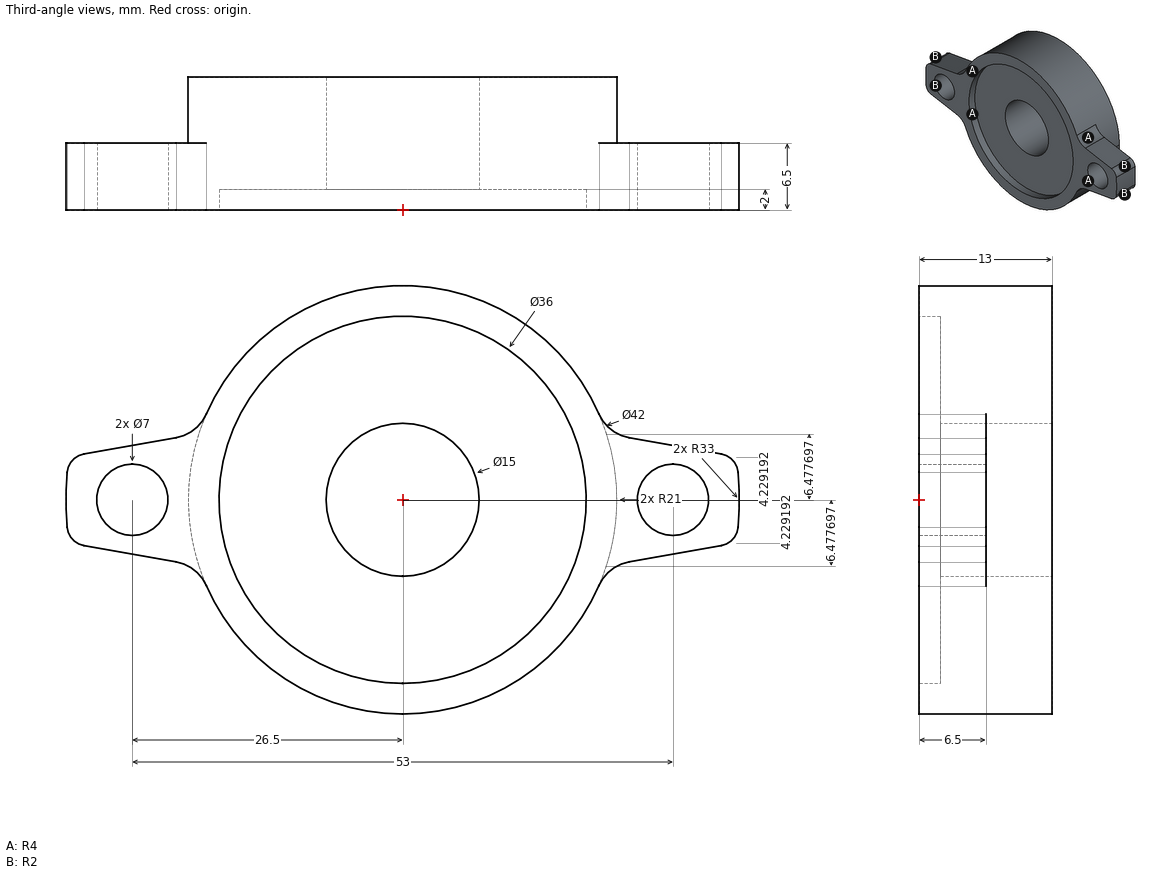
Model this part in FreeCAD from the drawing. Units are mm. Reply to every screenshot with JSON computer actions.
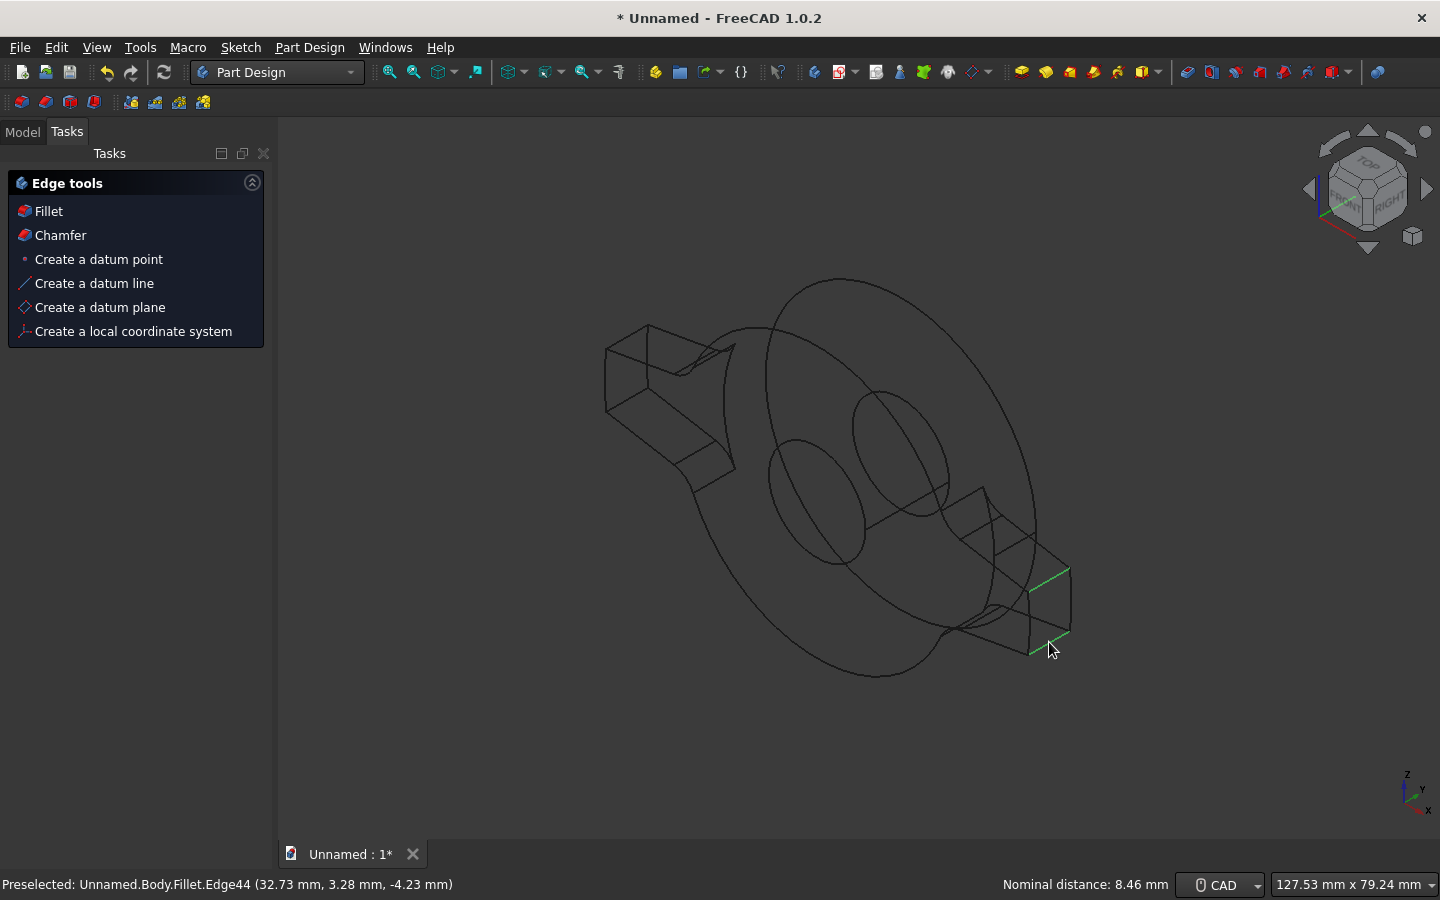
{"action": "left_click", "coordinate": [627, 399], "text": "ctrl"}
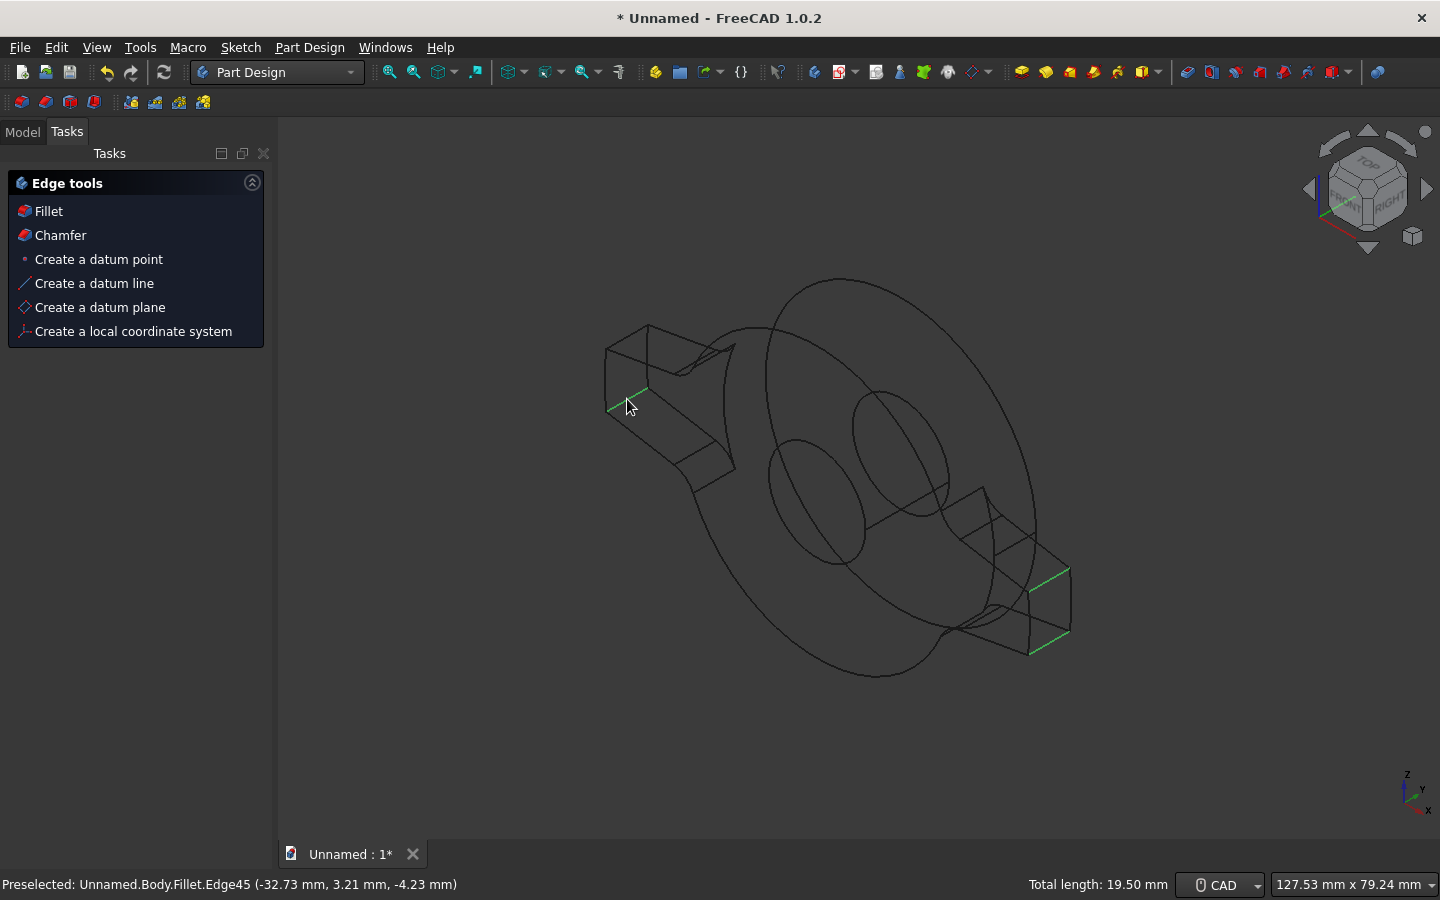
{"action": "left_click", "coordinate": [627, 336], "text": "ctrl"}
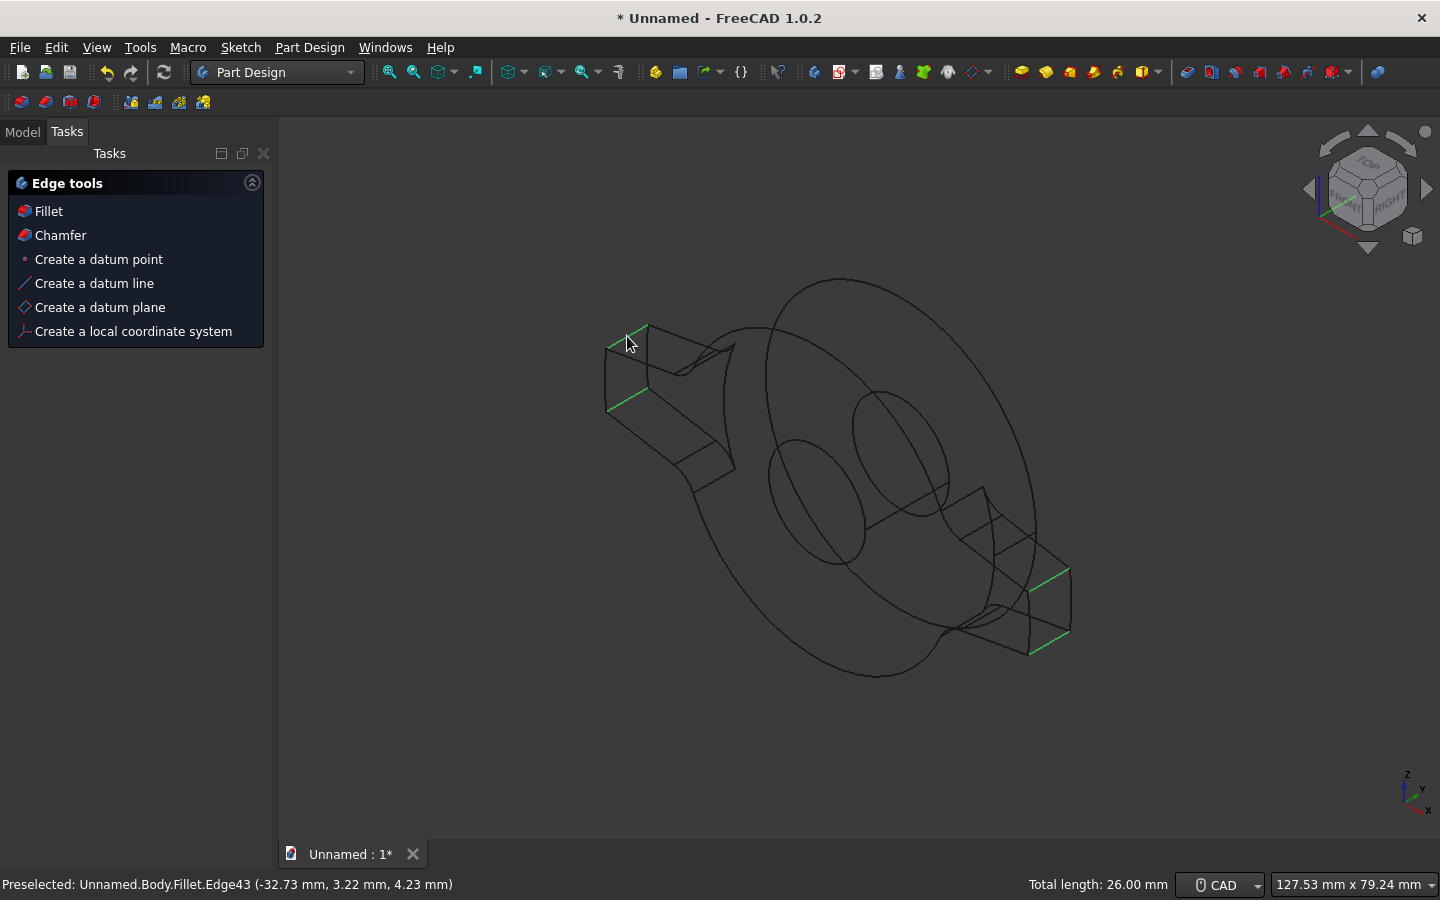
{"action": "key", "text": "v 1"}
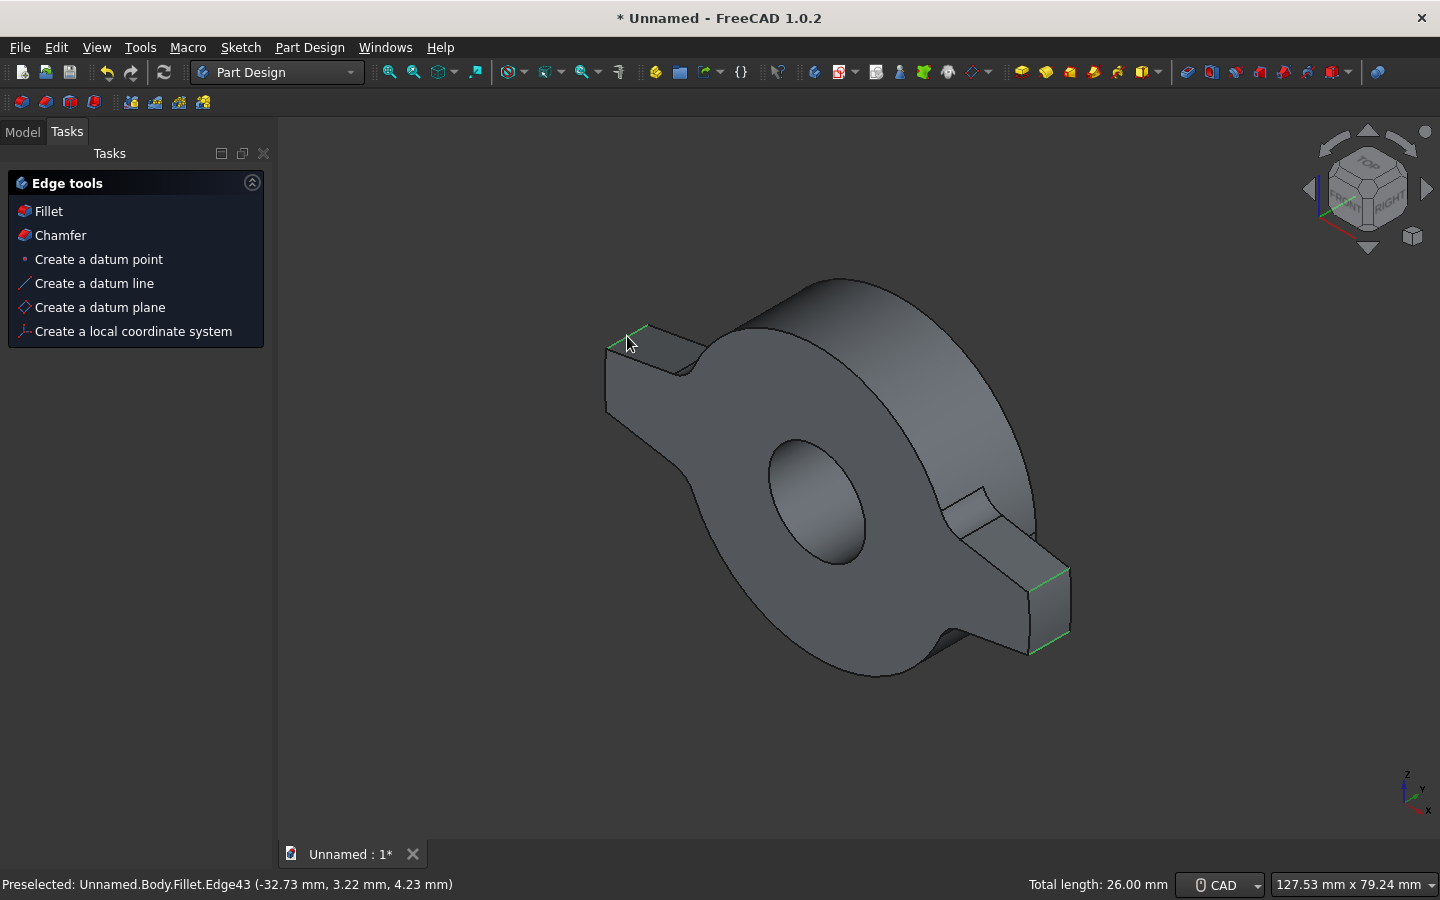
{"action": "left_click", "coordinate": [22, 102]}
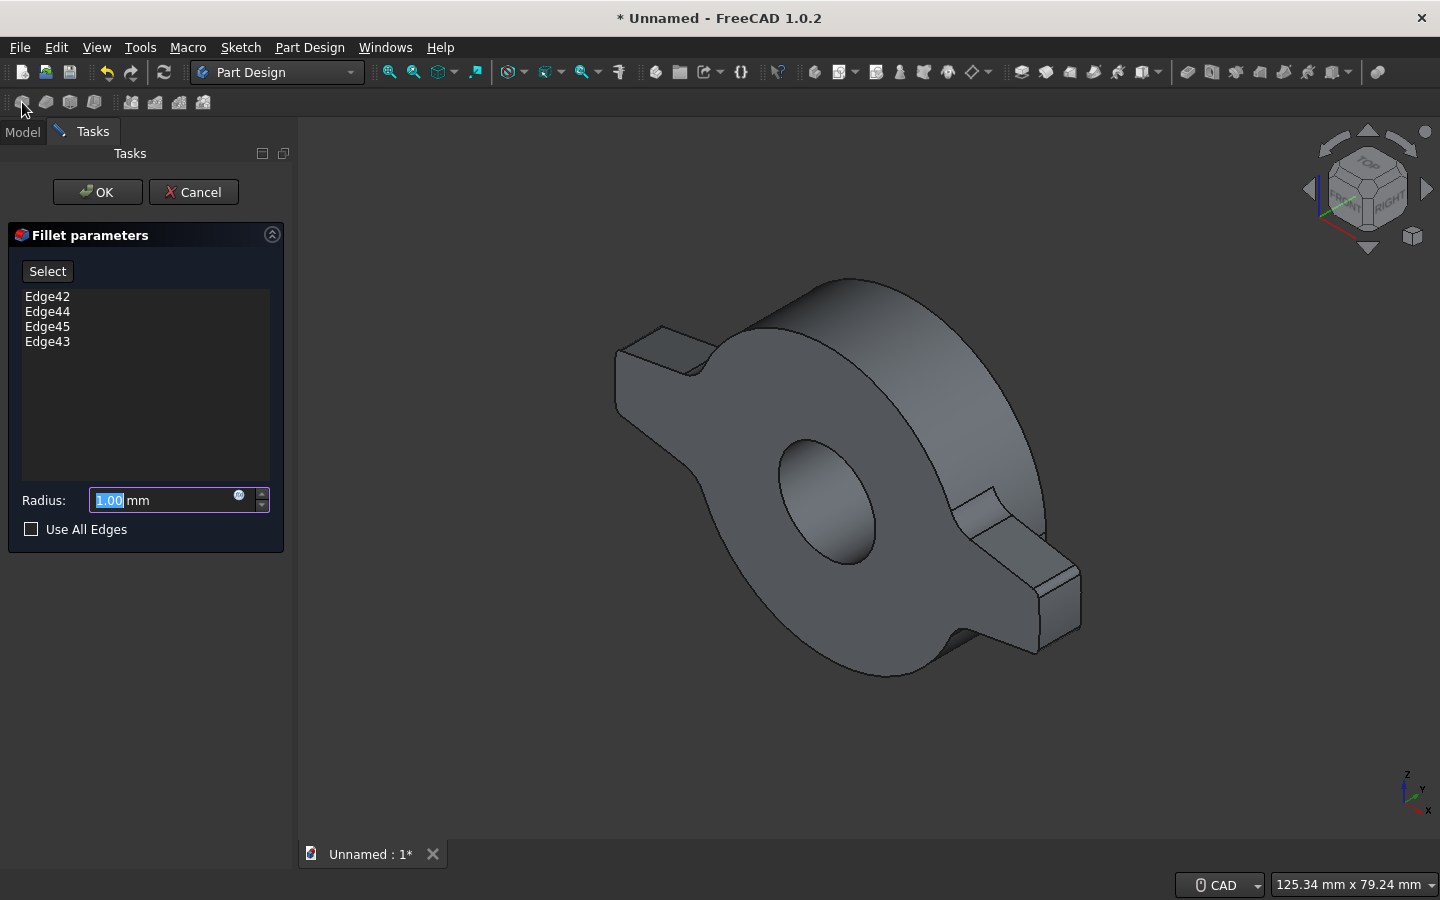
{"action": "type", "text": "2"}
{"action": "key", "text": "Tab"}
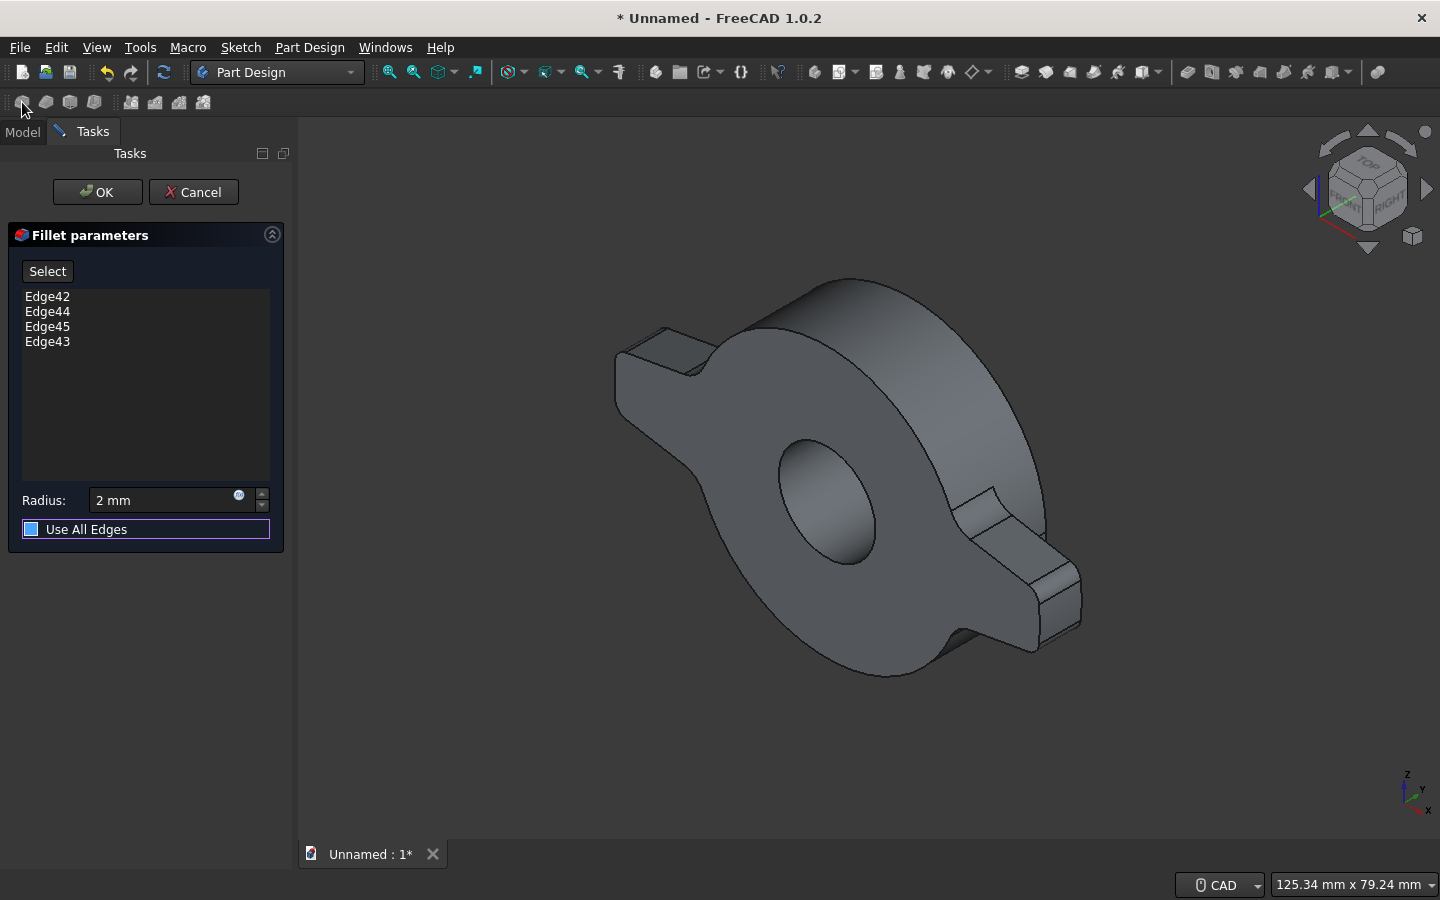
{"action": "left_click", "coordinate": [98, 192]}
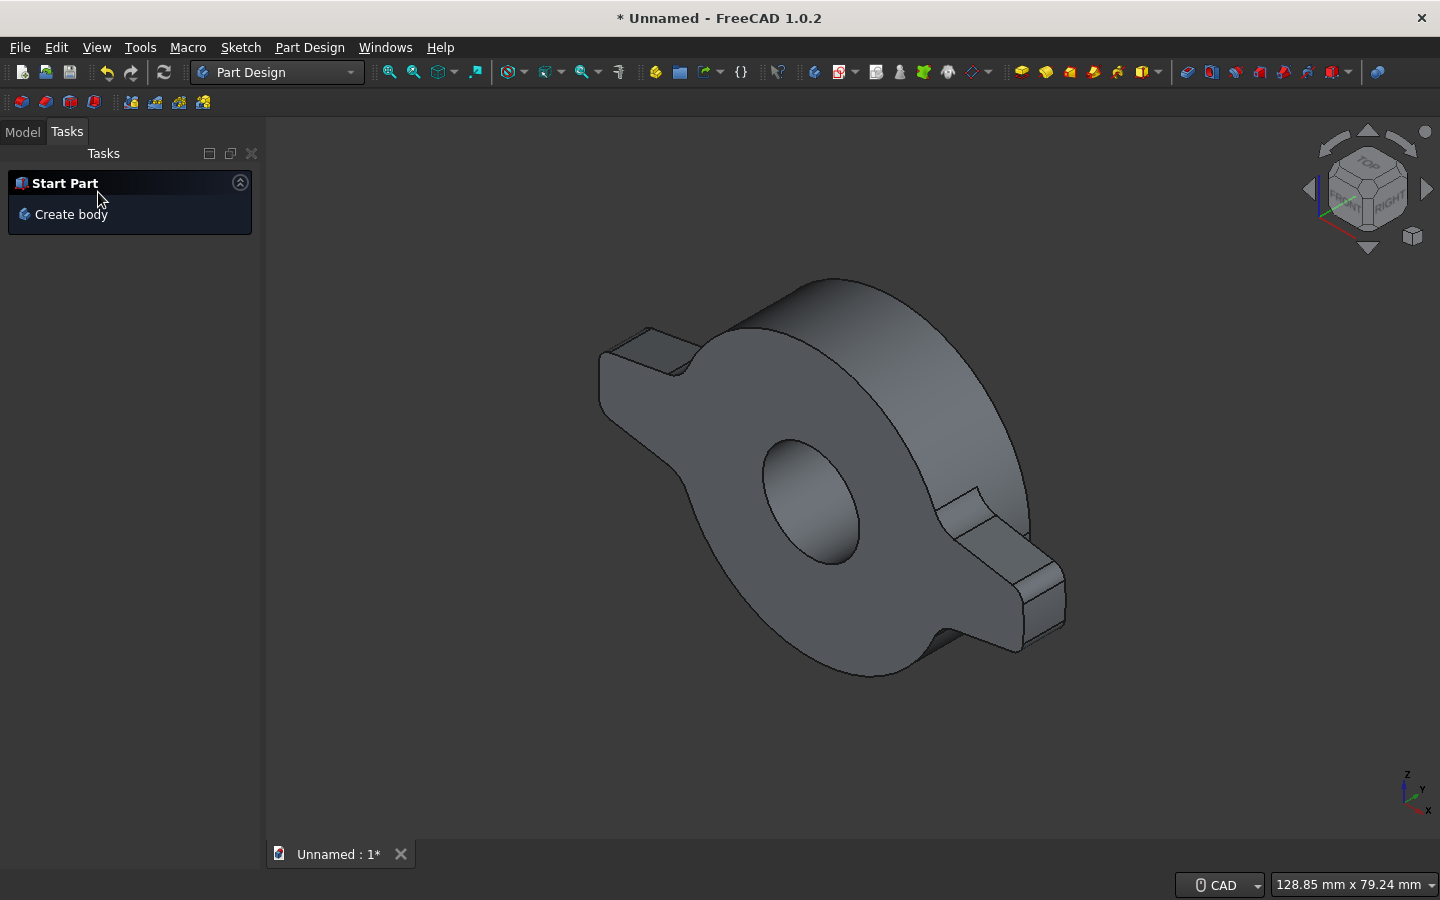
{"action": "key", "text": "4"}